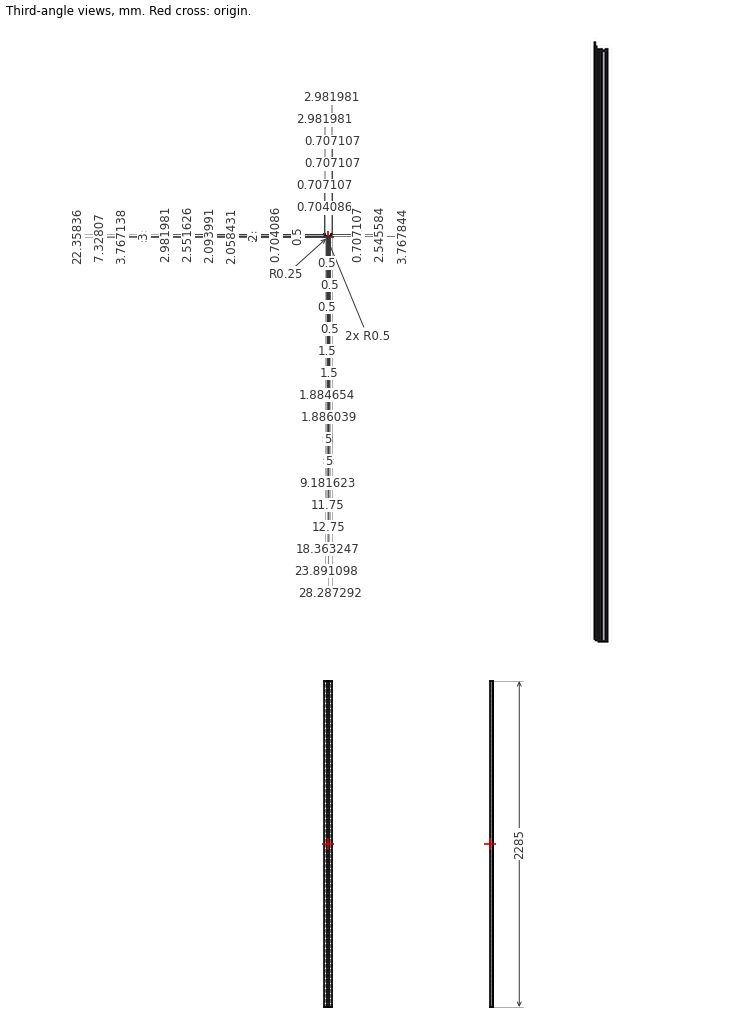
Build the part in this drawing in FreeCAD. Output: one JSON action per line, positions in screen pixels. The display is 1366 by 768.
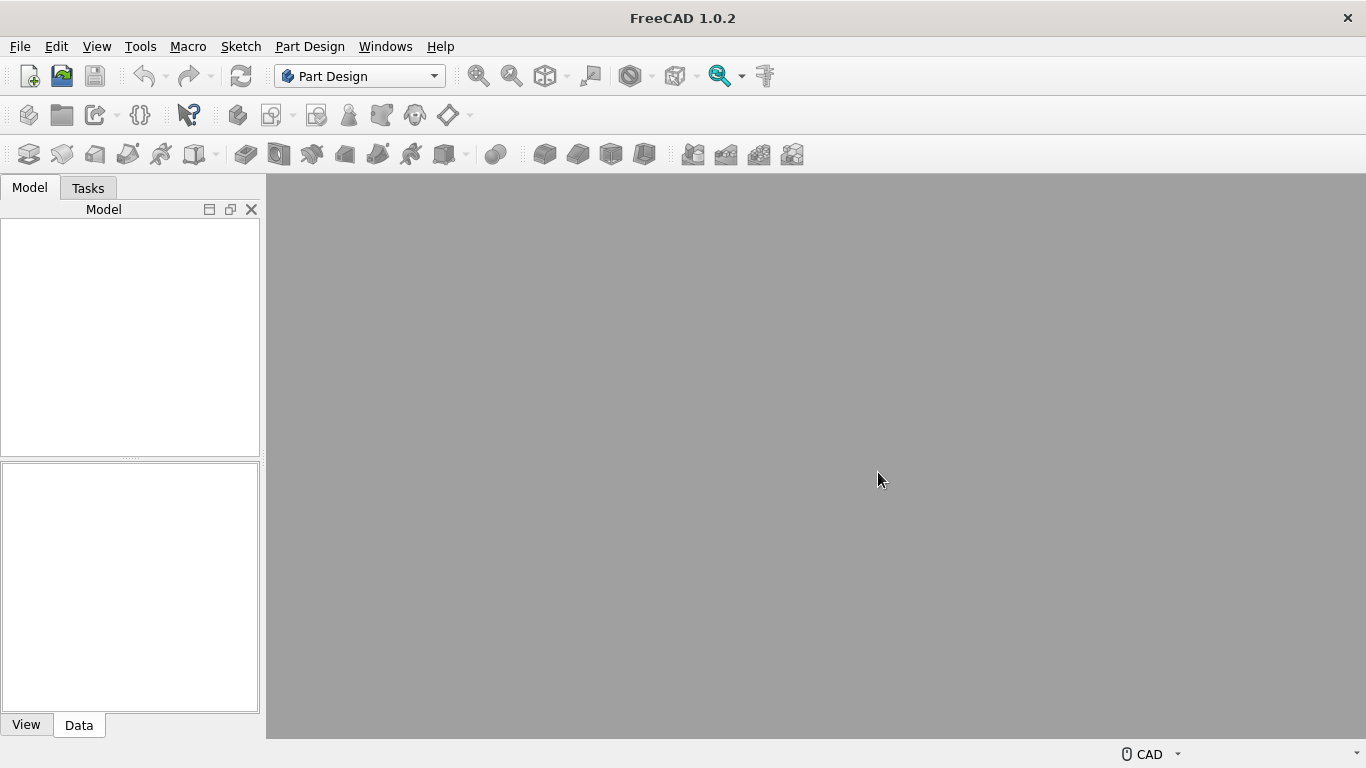
{"action": "left_click", "coordinate": [29, 76]}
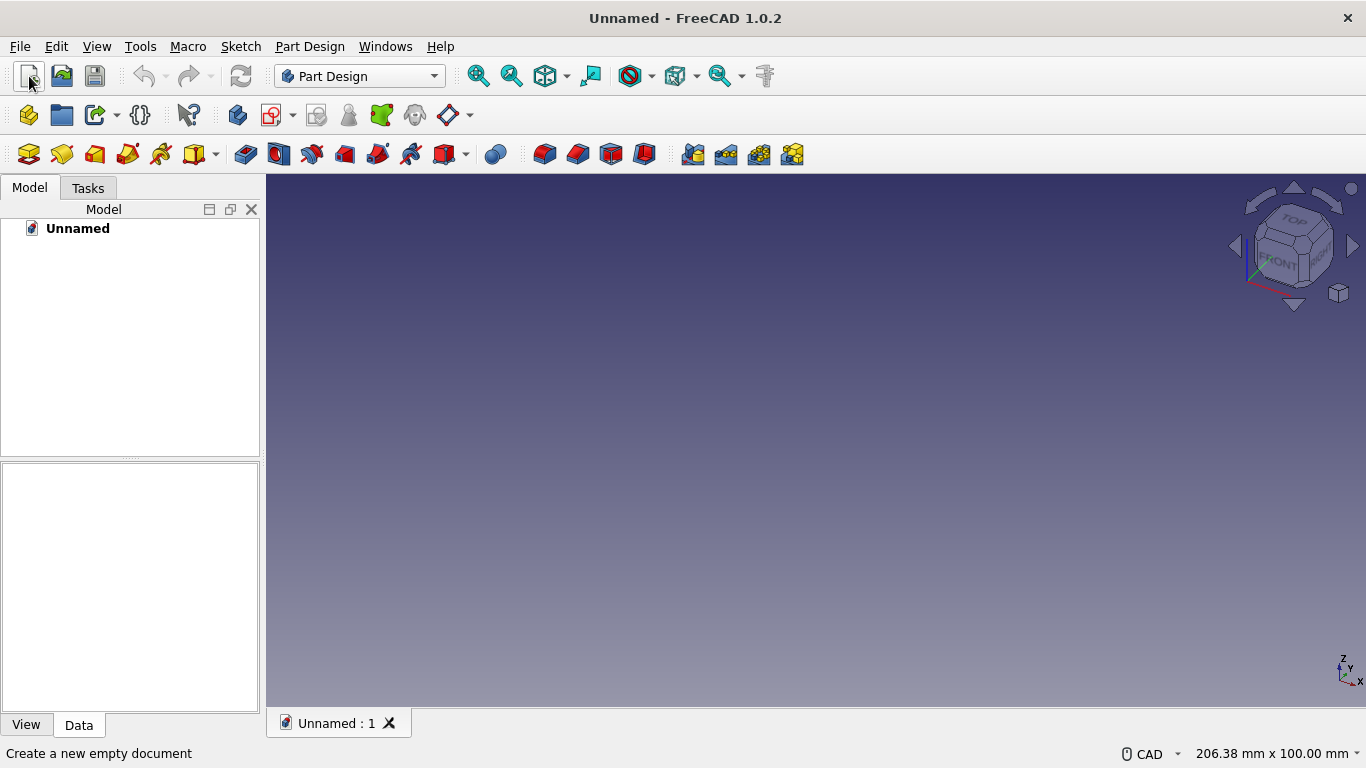
{"action": "left_click", "coordinate": [270, 116]}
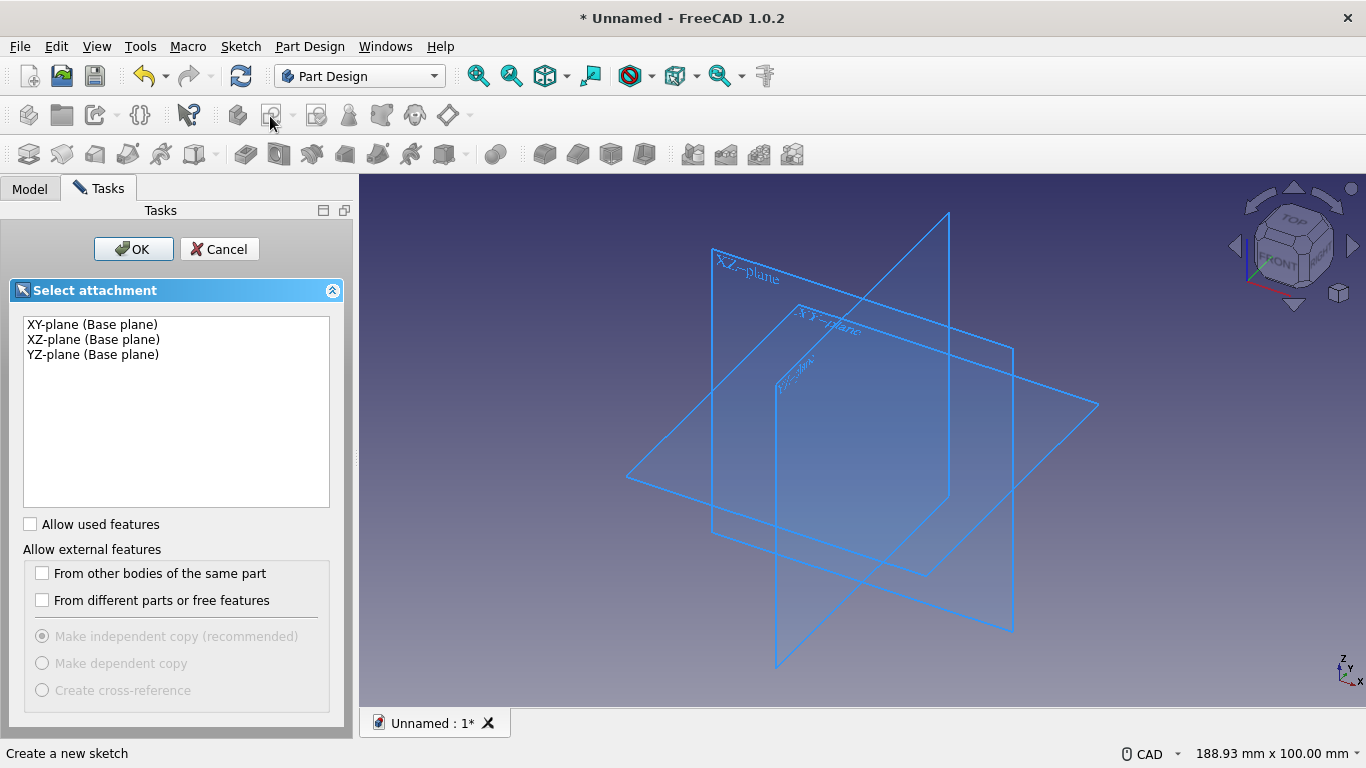
{"action": "left_click", "coordinate": [84, 324]}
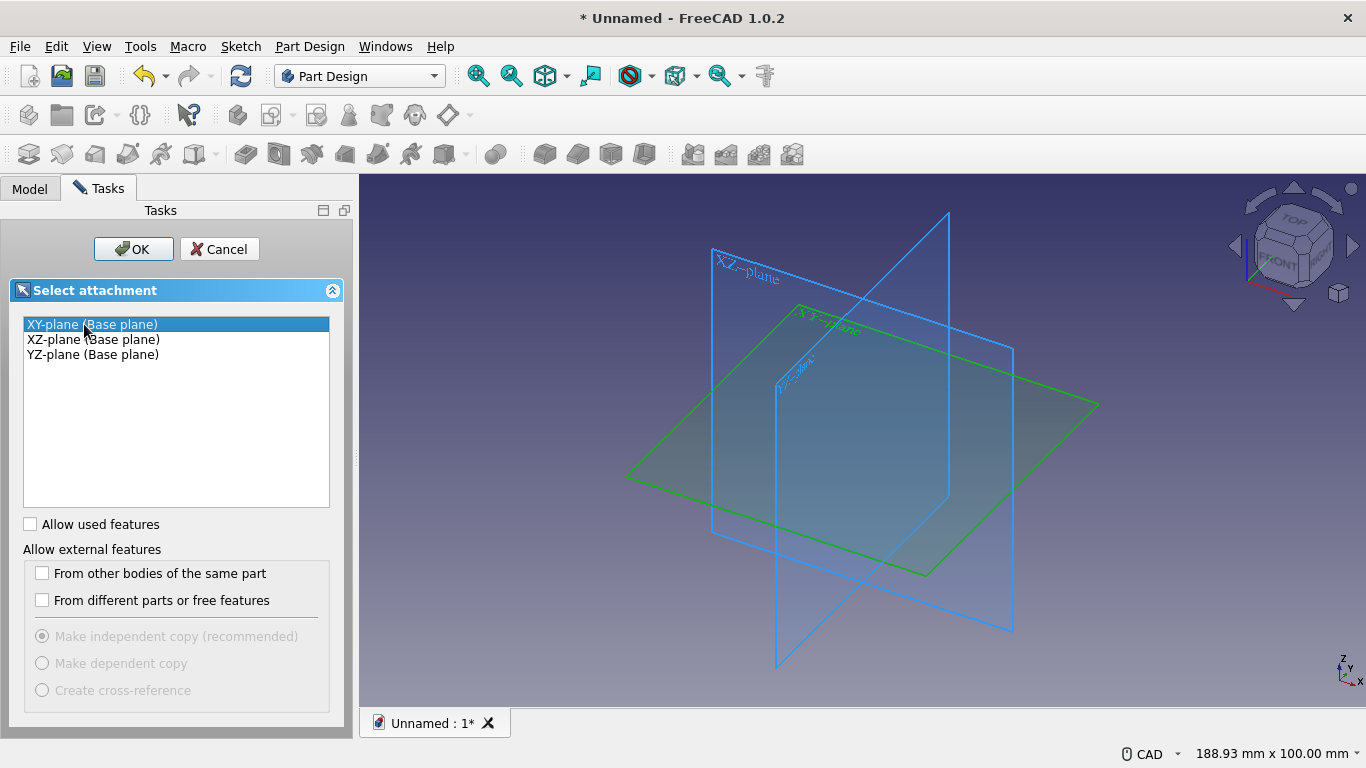
{"action": "left_click", "coordinate": [134, 249]}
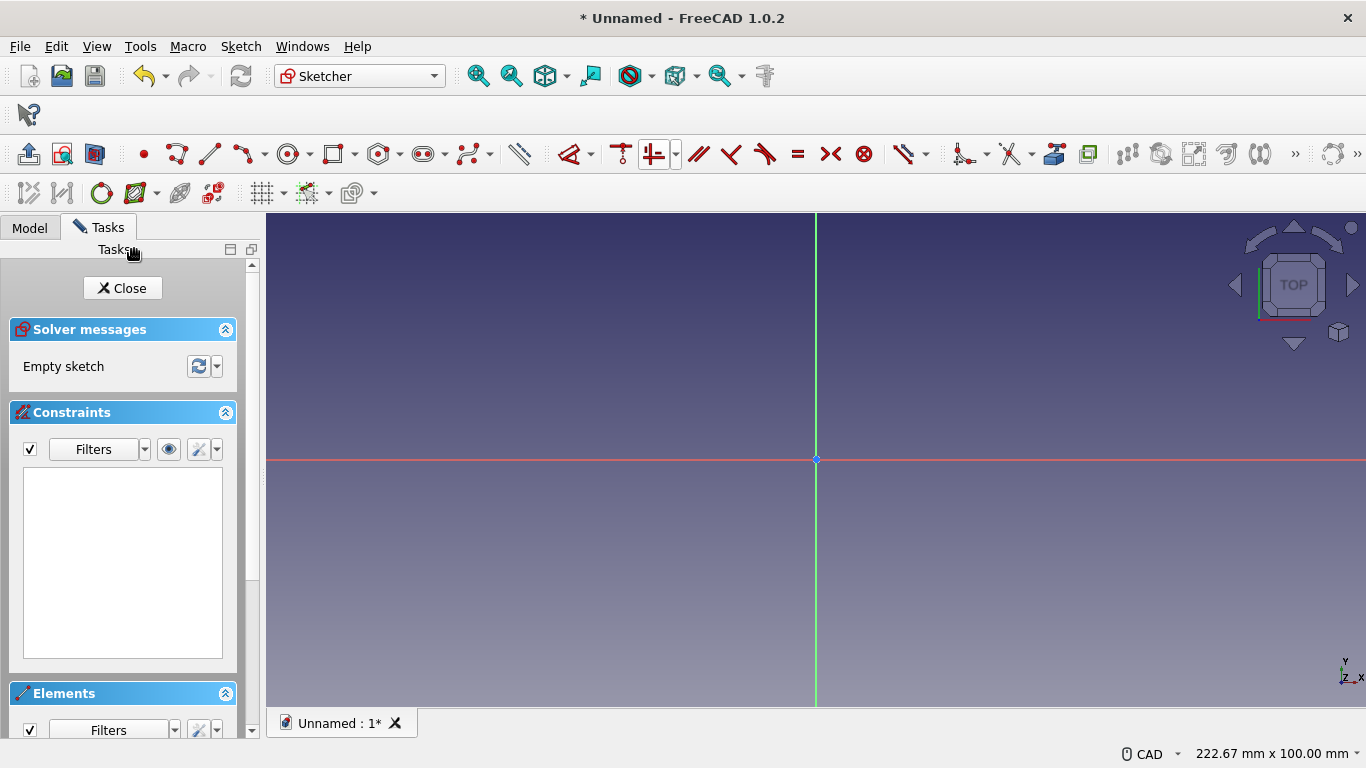
{"action": "scroll", "coordinate": [872, 360], "scroll_direction": "up", "scroll_amount": 4}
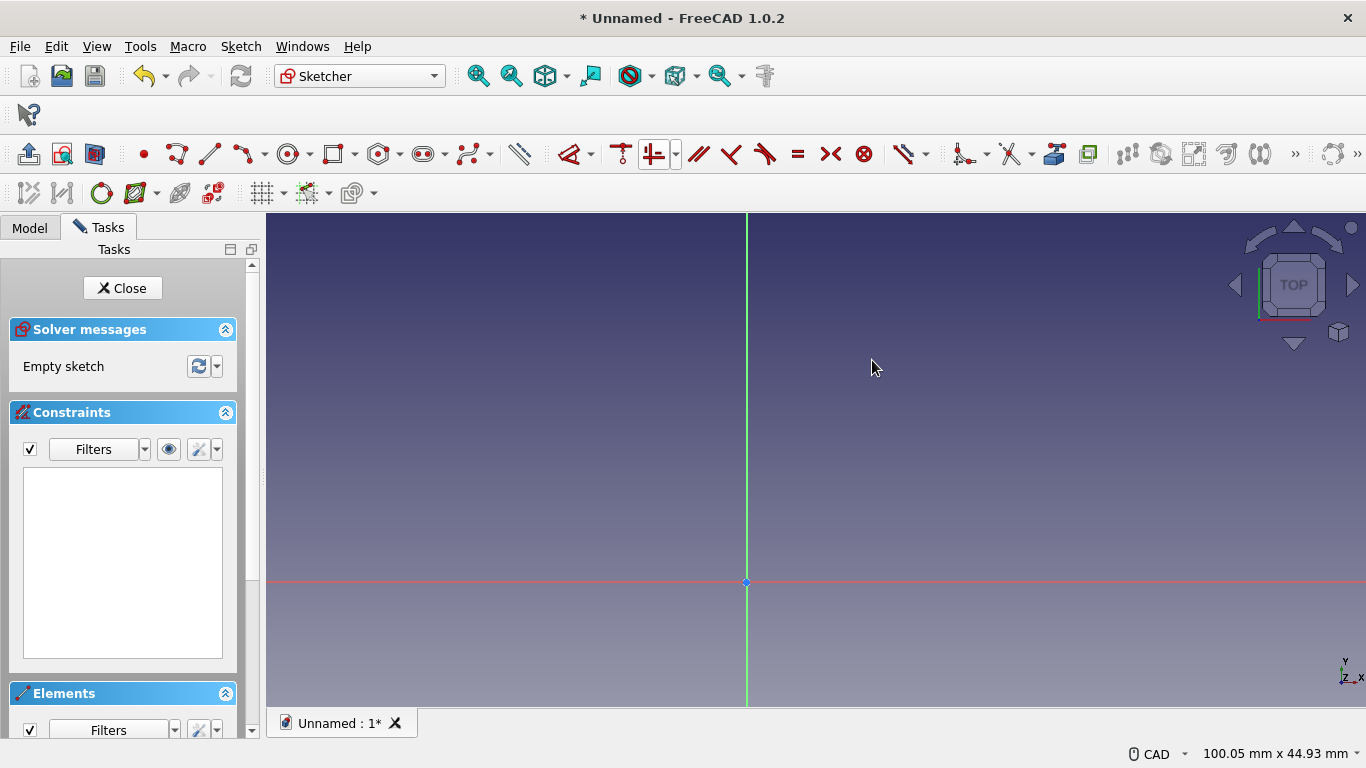
{"action": "left_click", "coordinate": [177, 154]}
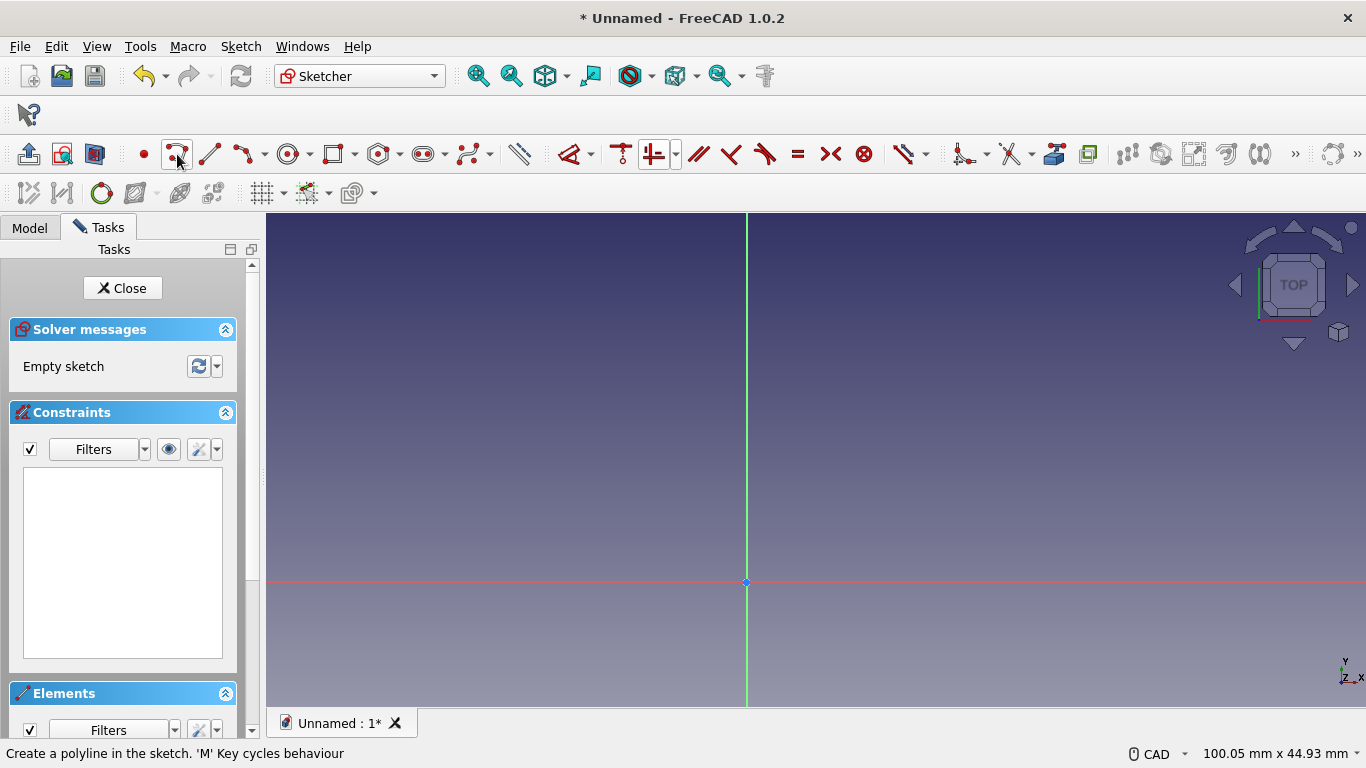
{"action": "scroll", "coordinate": [744, 560], "scroll_direction": "up", "scroll_amount": 9}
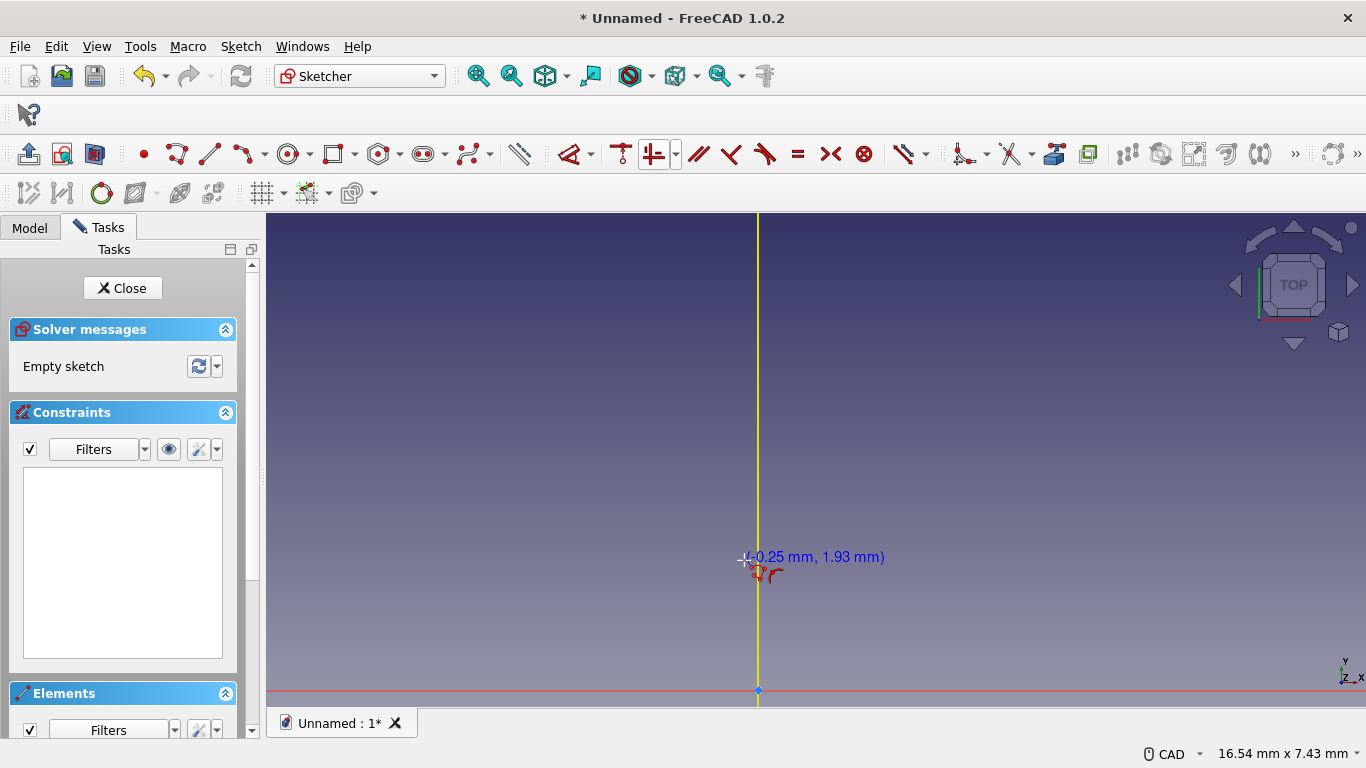
{"action": "left_click", "coordinate": [741, 558]}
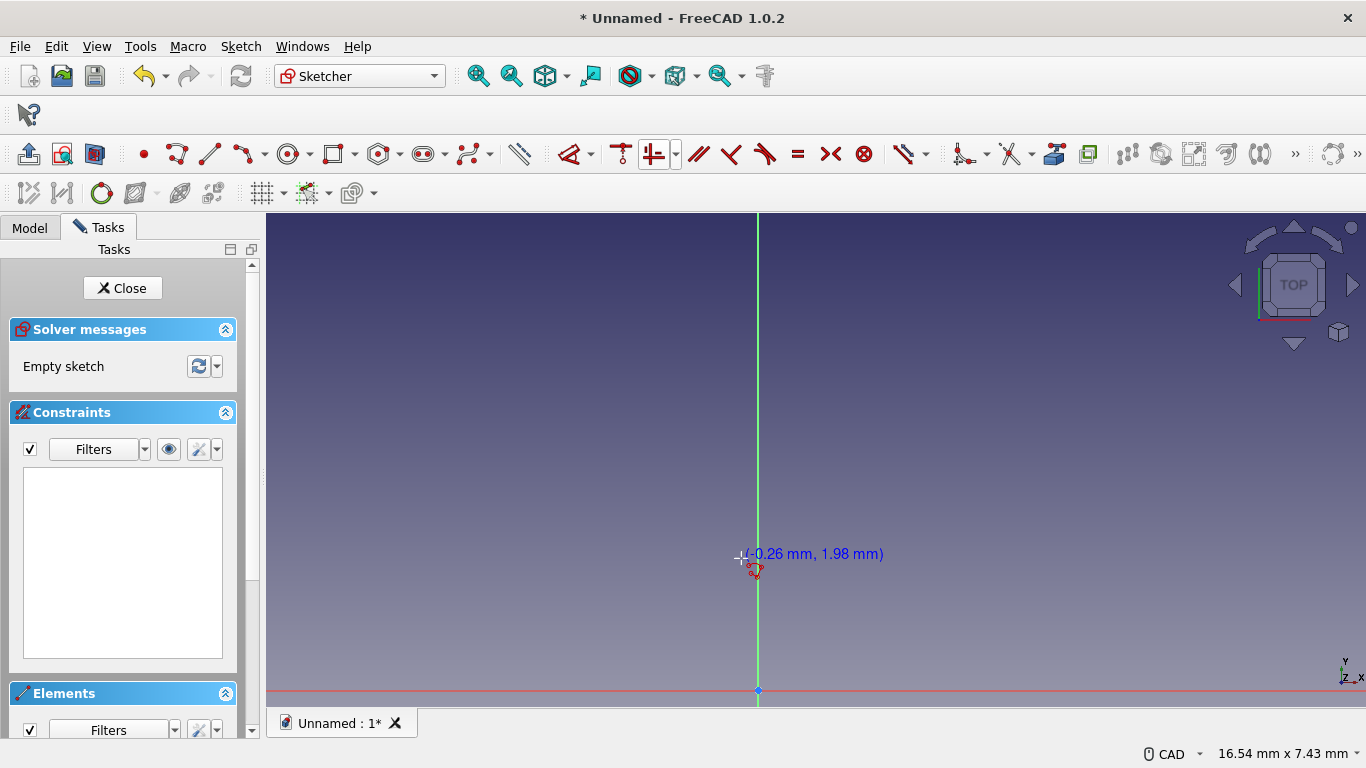
{"action": "scroll", "coordinate": [745, 562], "scroll_direction": "down", "scroll_amount": 9}